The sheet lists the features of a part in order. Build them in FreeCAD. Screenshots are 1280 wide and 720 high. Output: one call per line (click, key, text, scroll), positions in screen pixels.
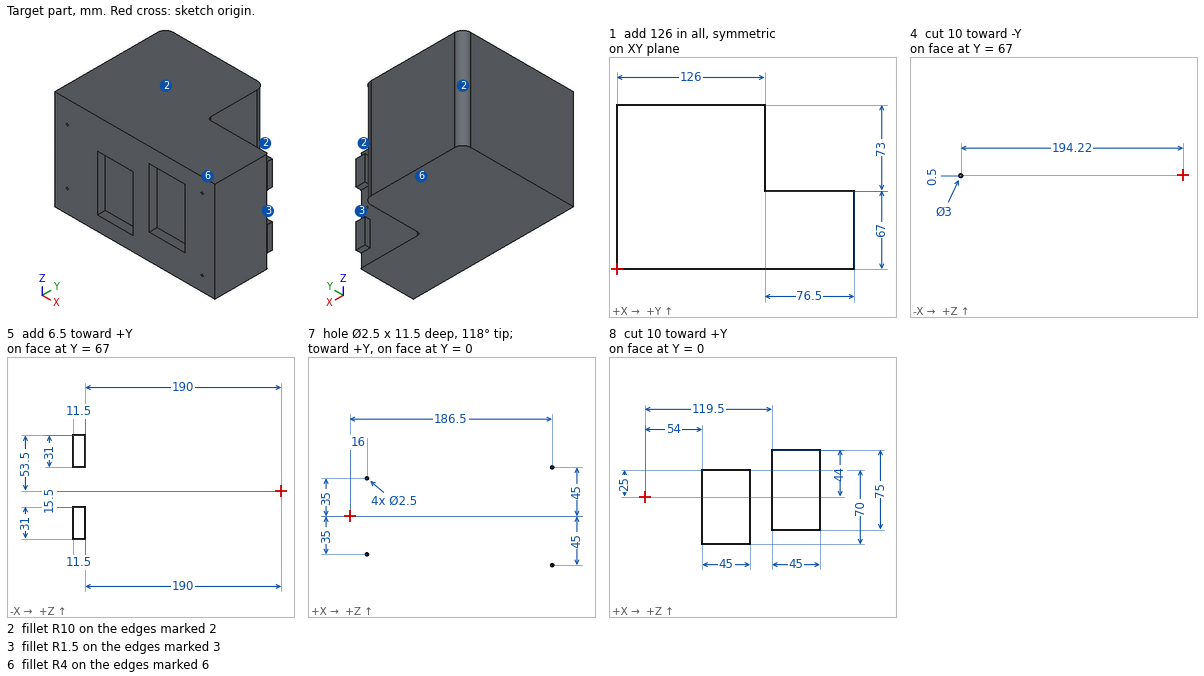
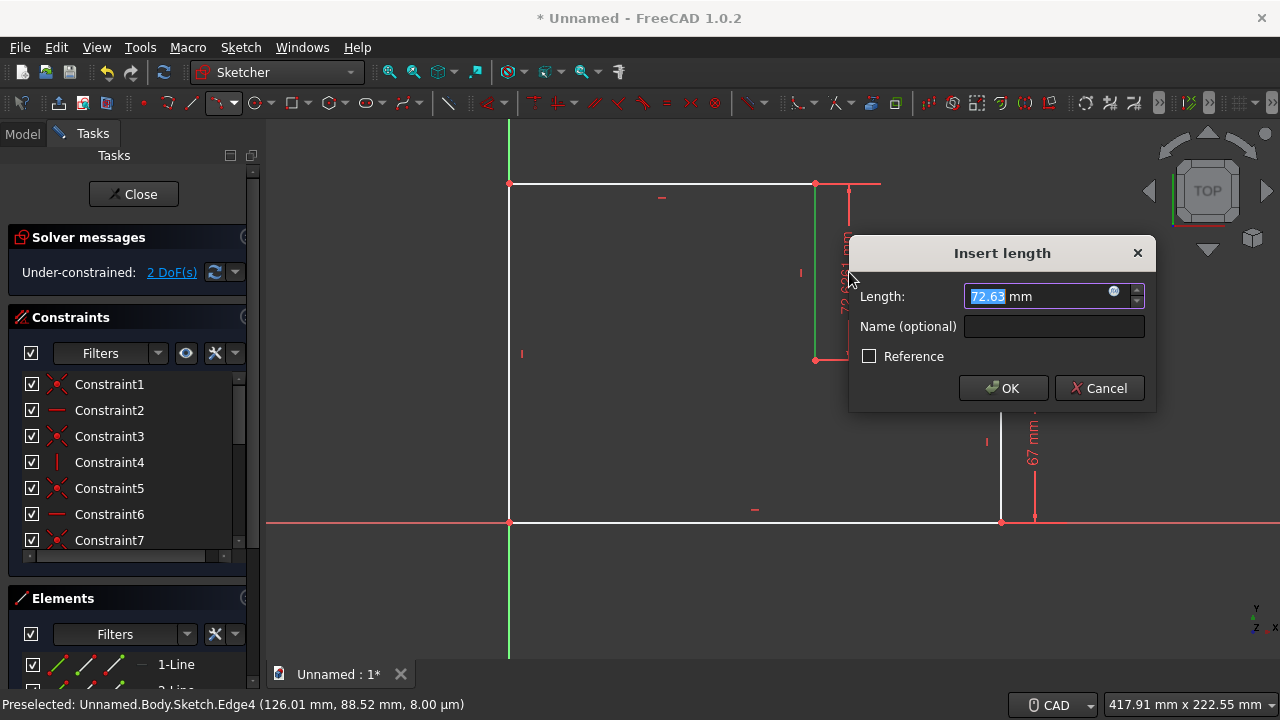
text(73)
key(Return)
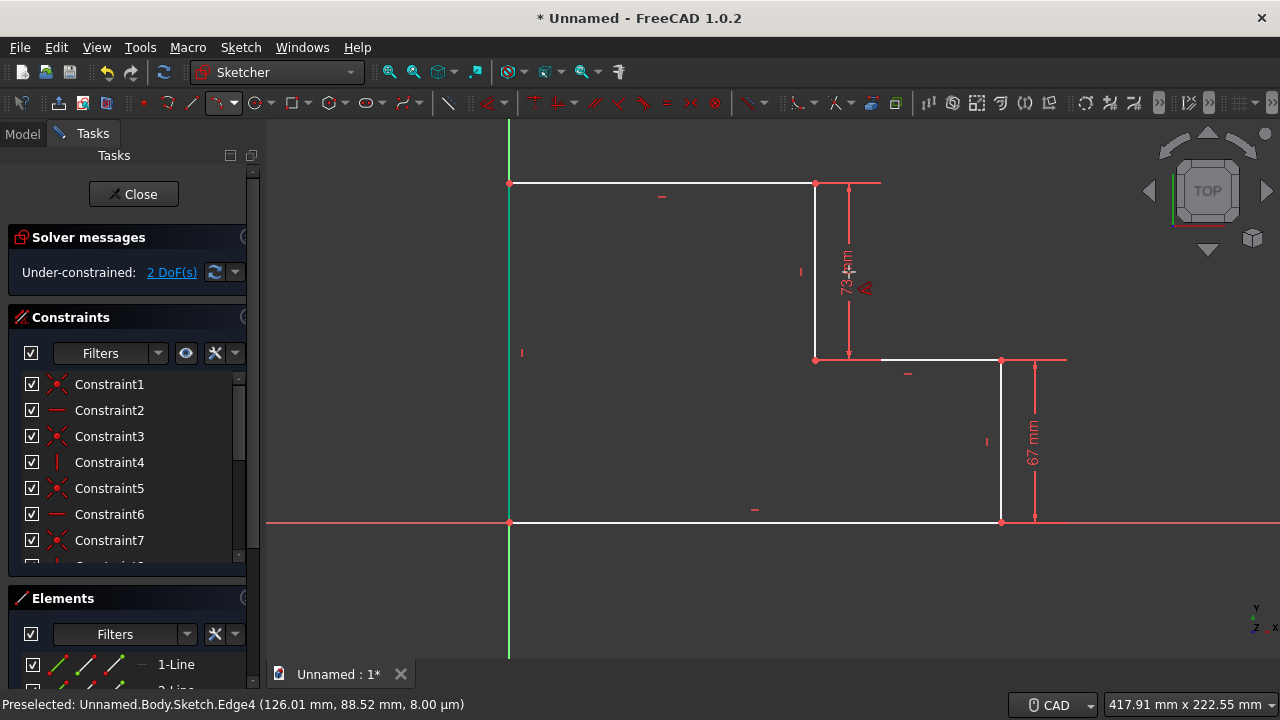
click(723, 183)
click(662, 149)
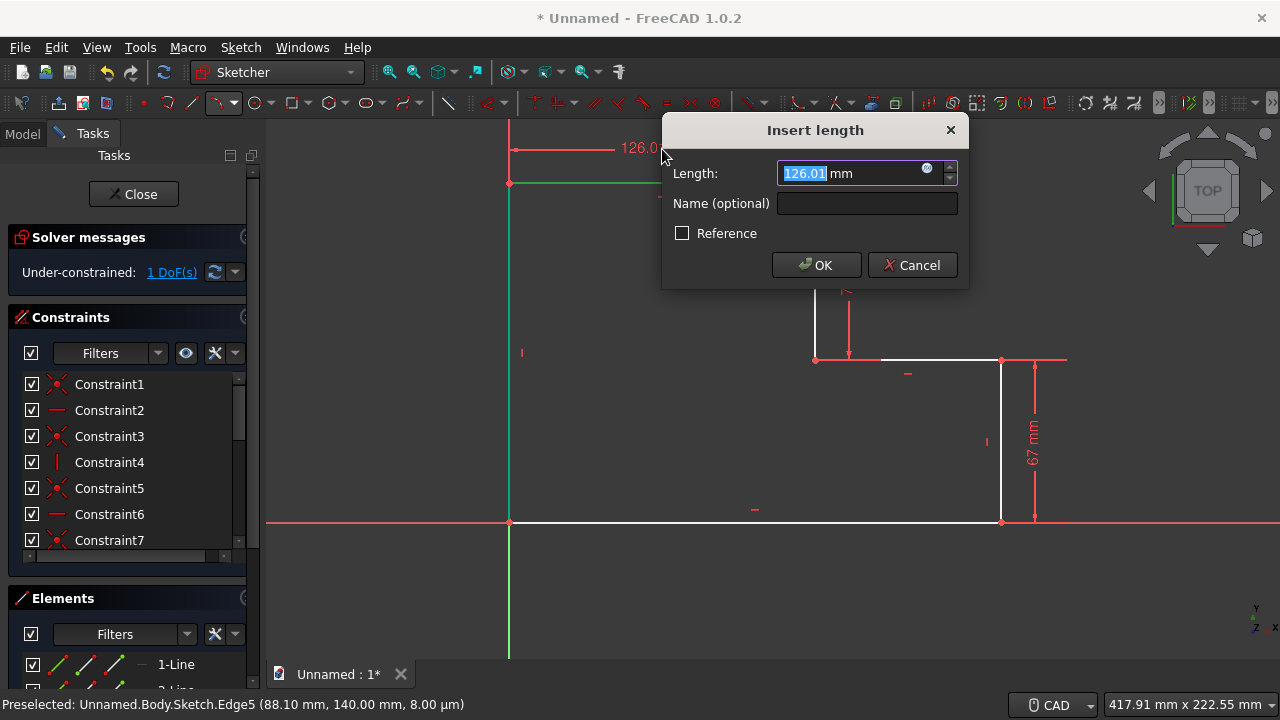
text(126)
key(Return)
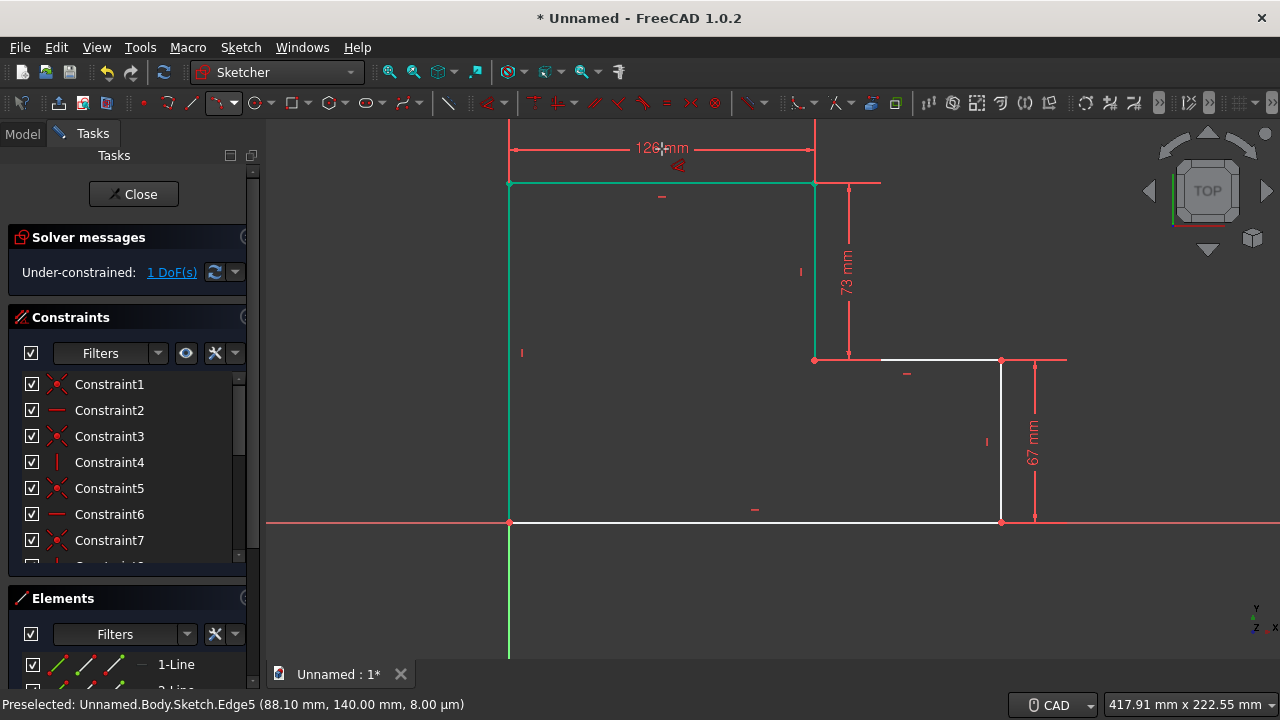
click(945, 360)
click(908, 394)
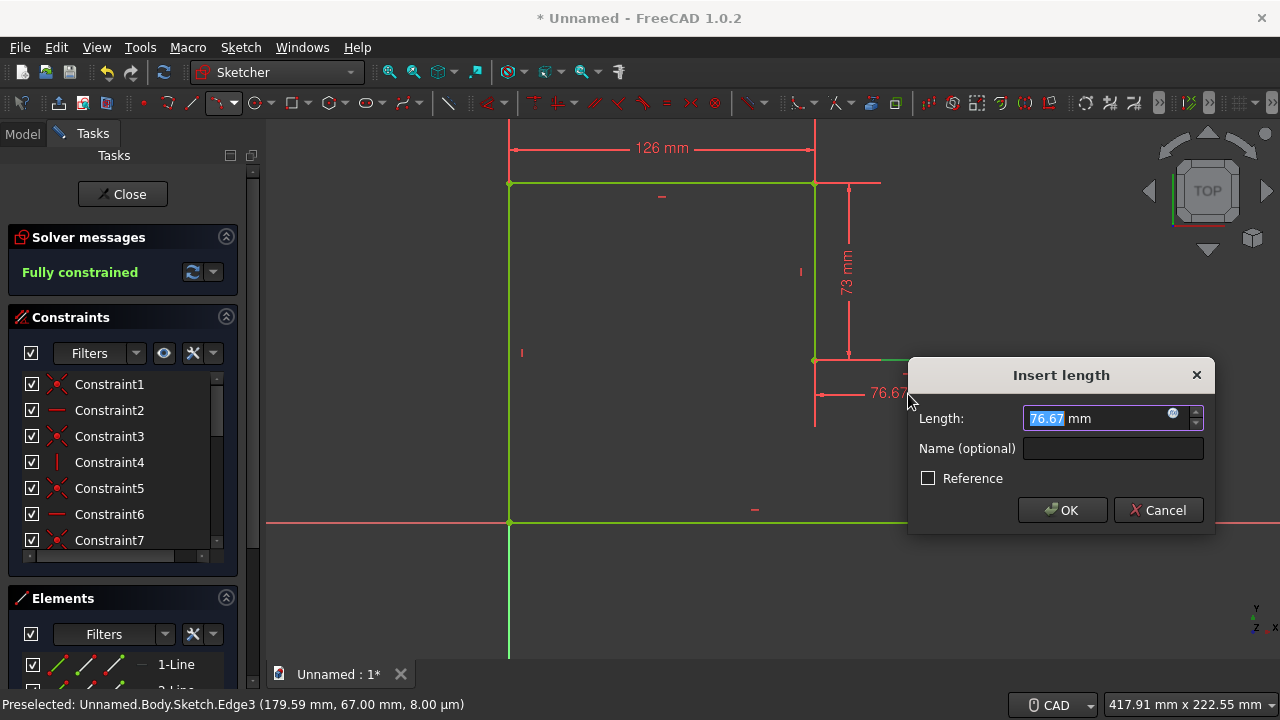
text(76.5)
key(Return)
key(Escape)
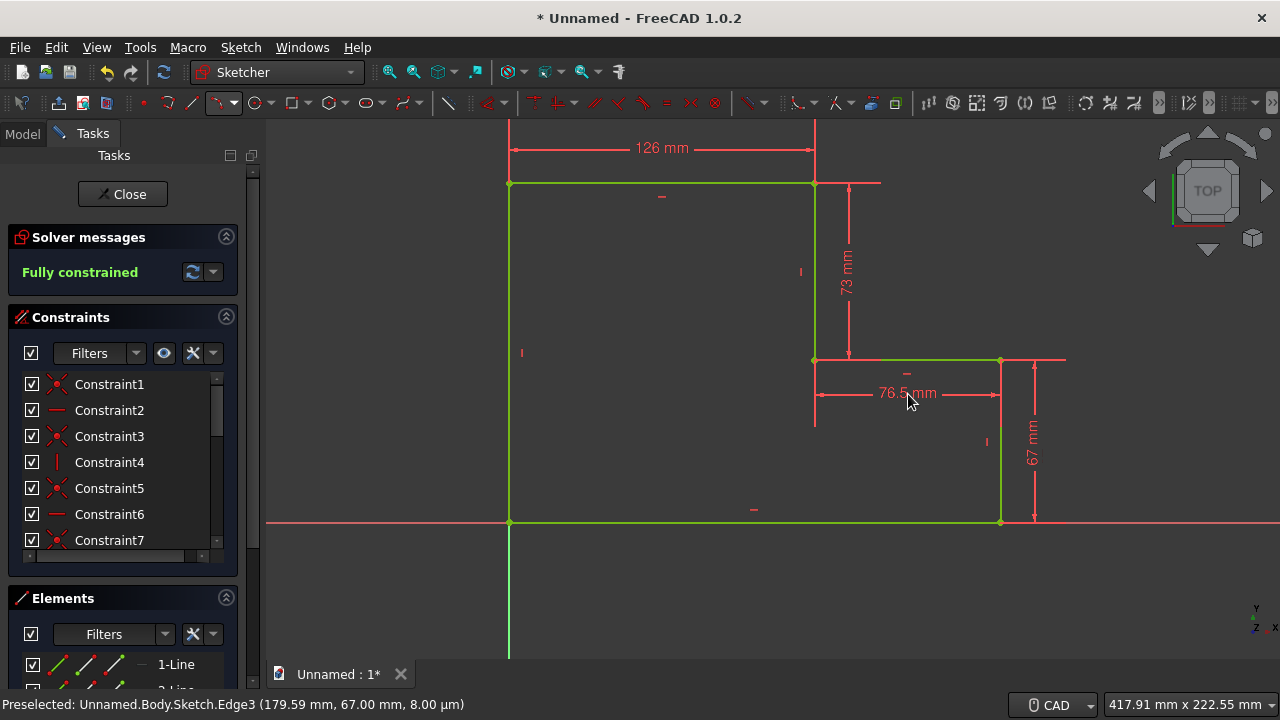
click(123, 194)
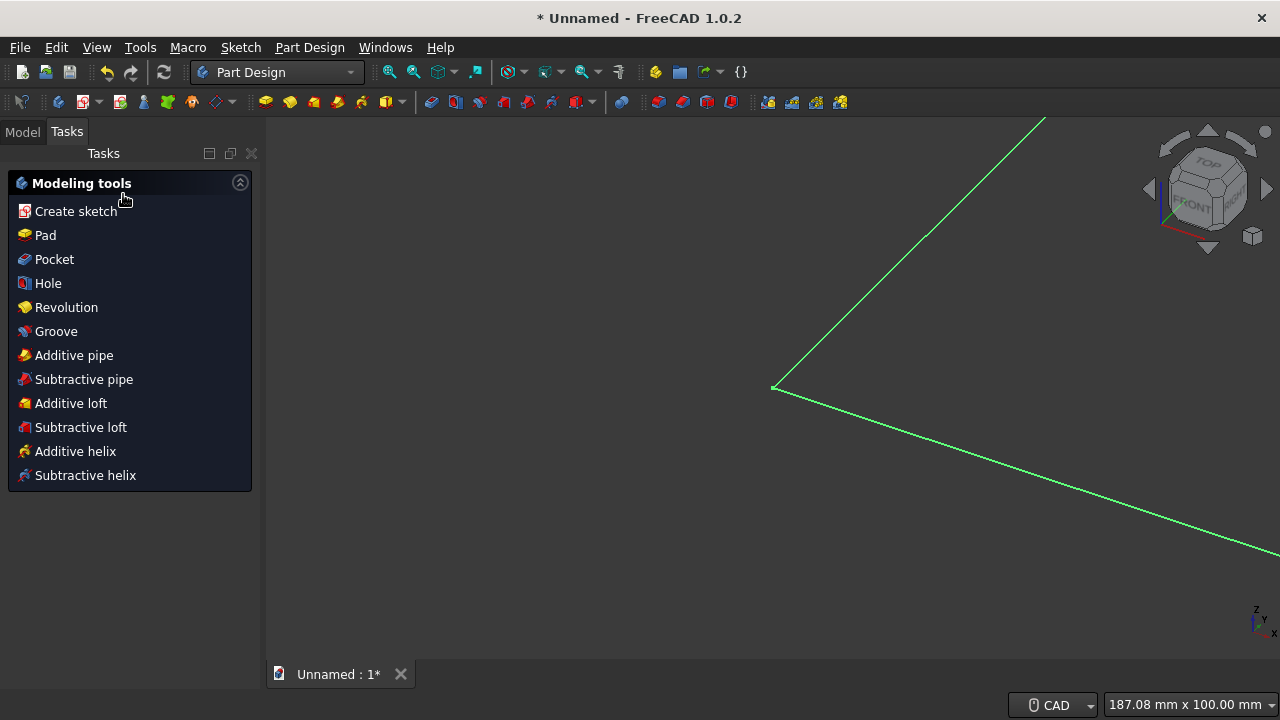
click(266, 102)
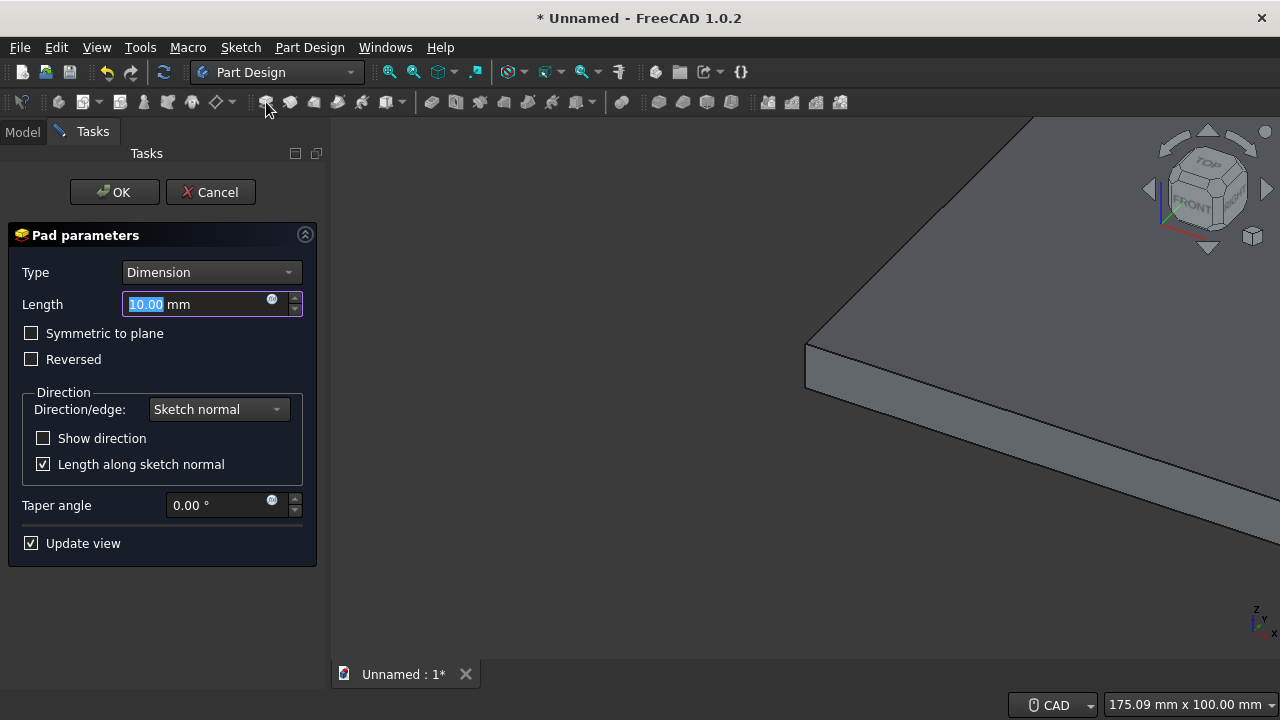
text(126)
key(Tab)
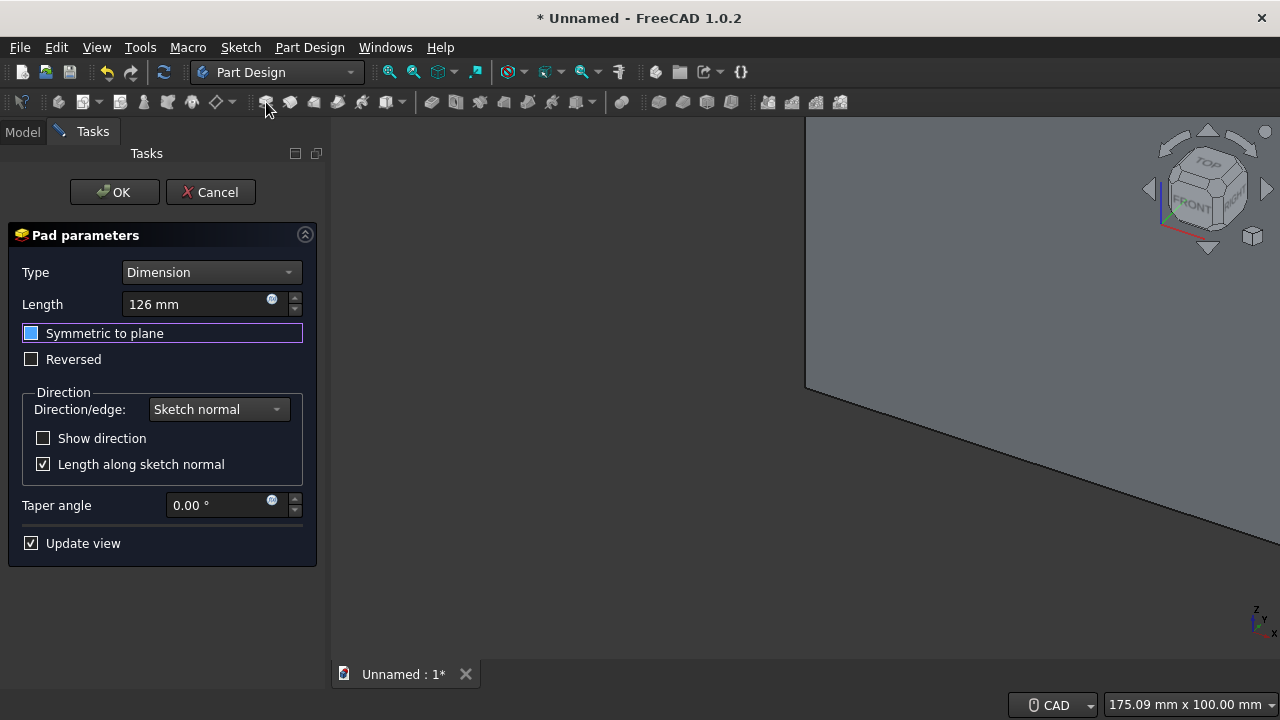
click(30, 333)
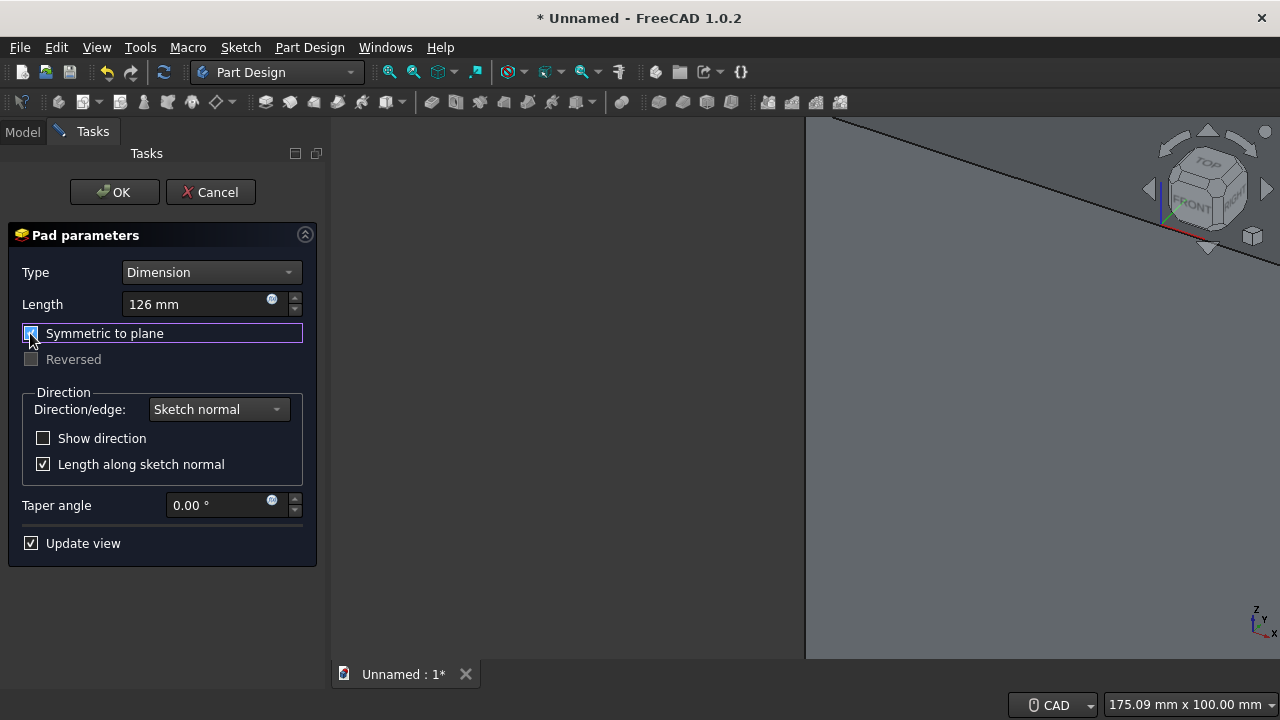
click(115, 192)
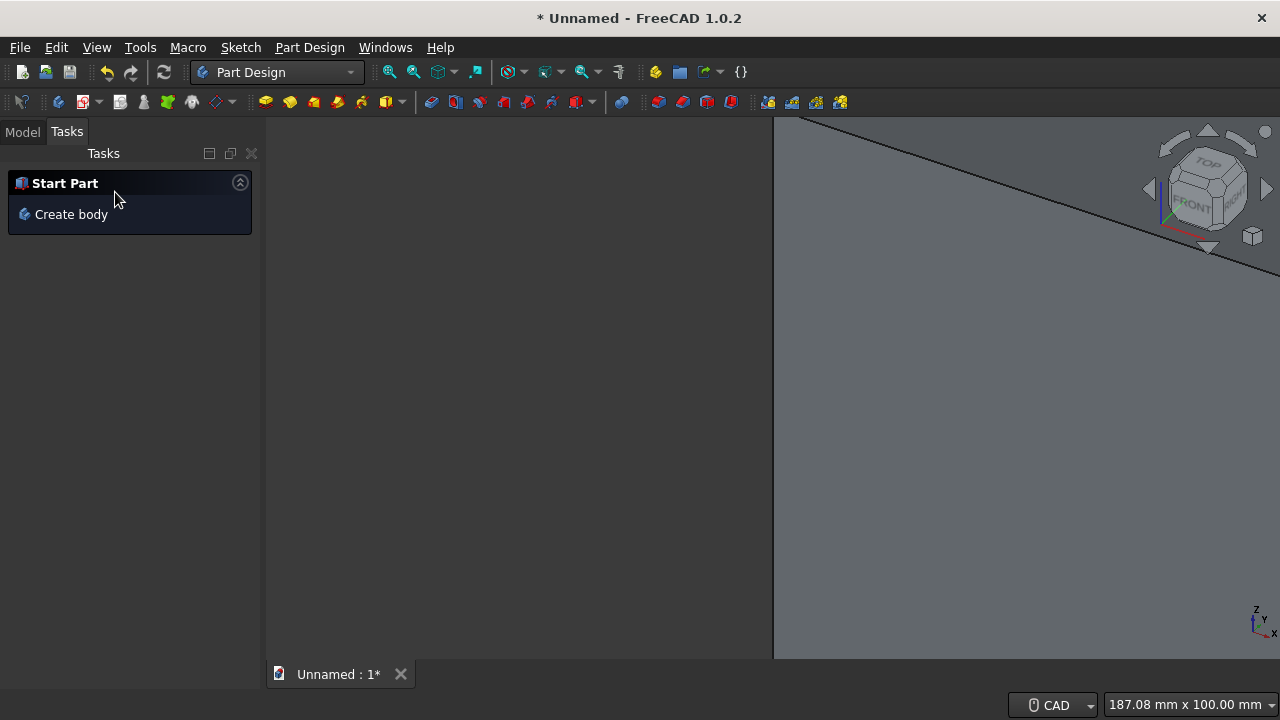
key(v)
key(f)